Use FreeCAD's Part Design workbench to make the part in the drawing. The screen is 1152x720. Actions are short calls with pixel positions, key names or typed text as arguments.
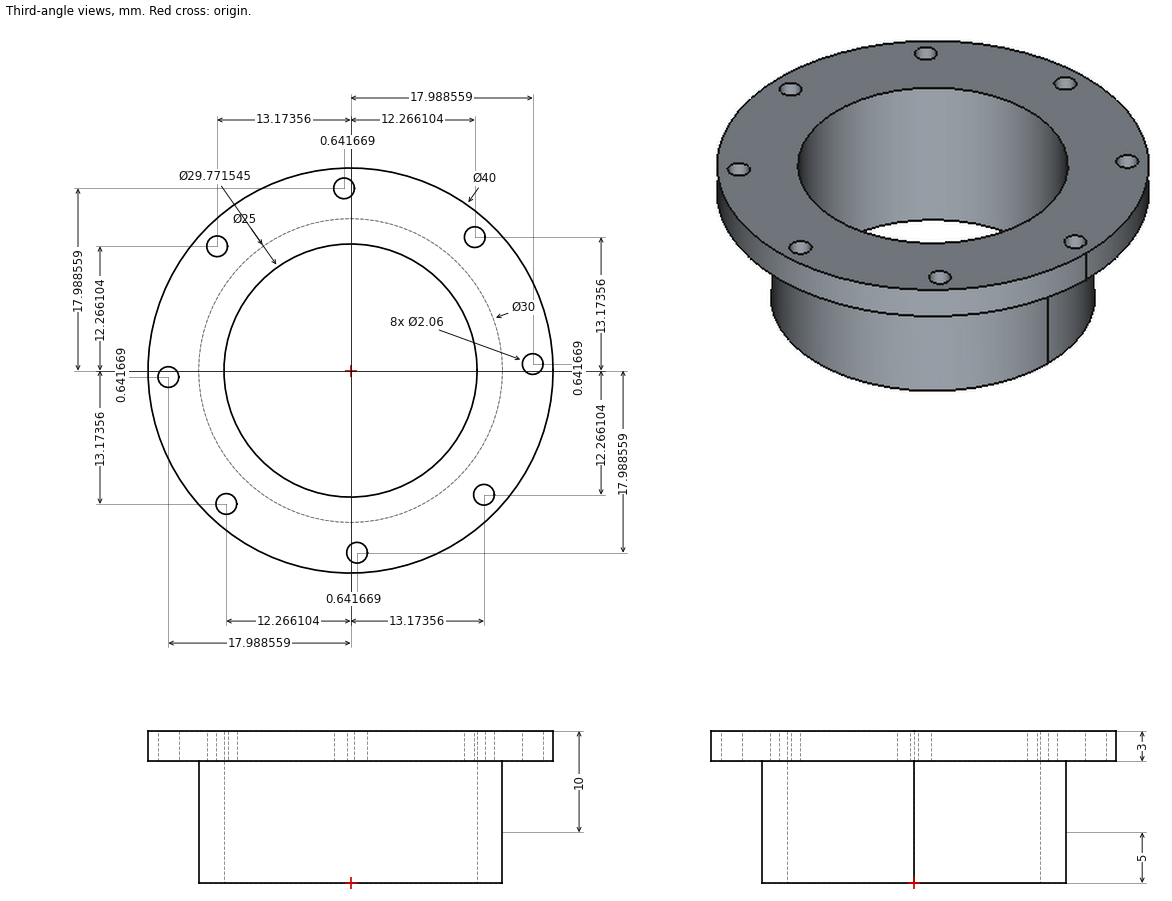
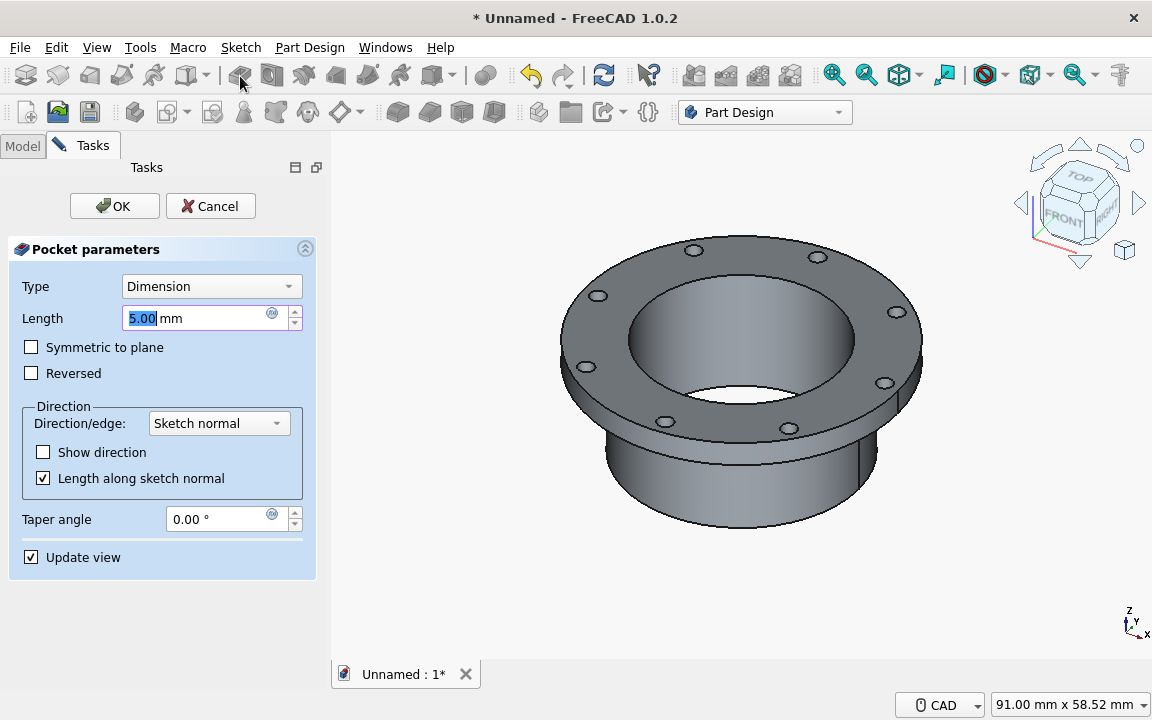
text(10)
key(Tab)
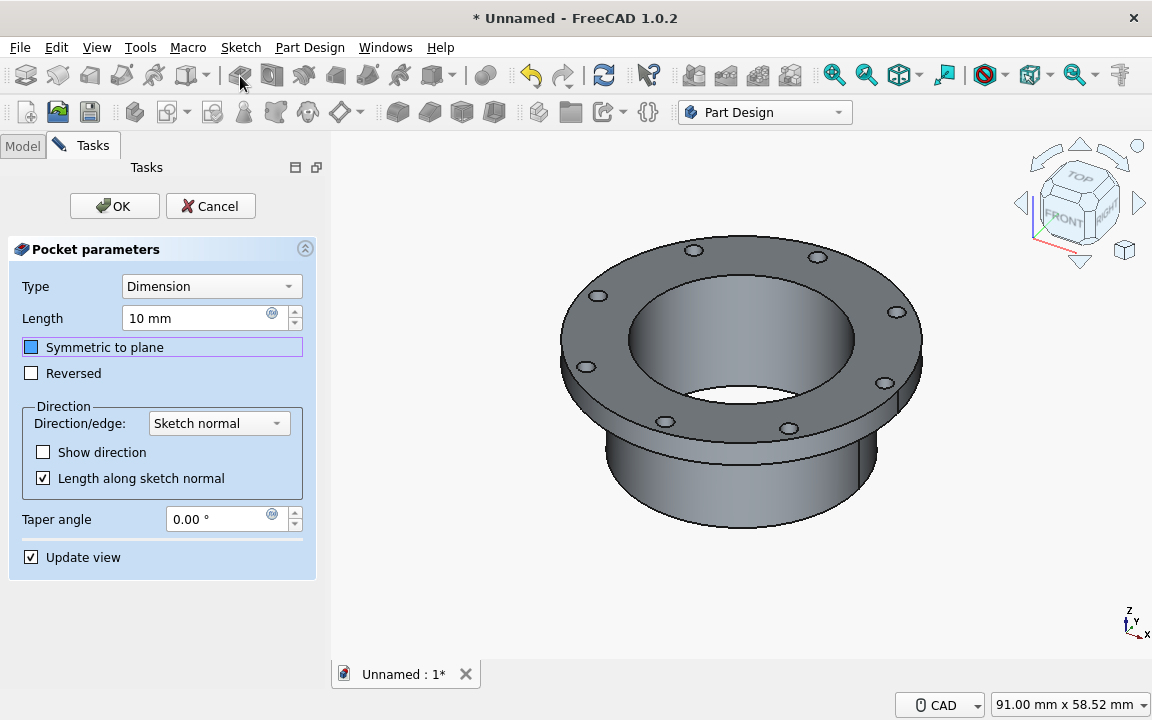
click(115, 206)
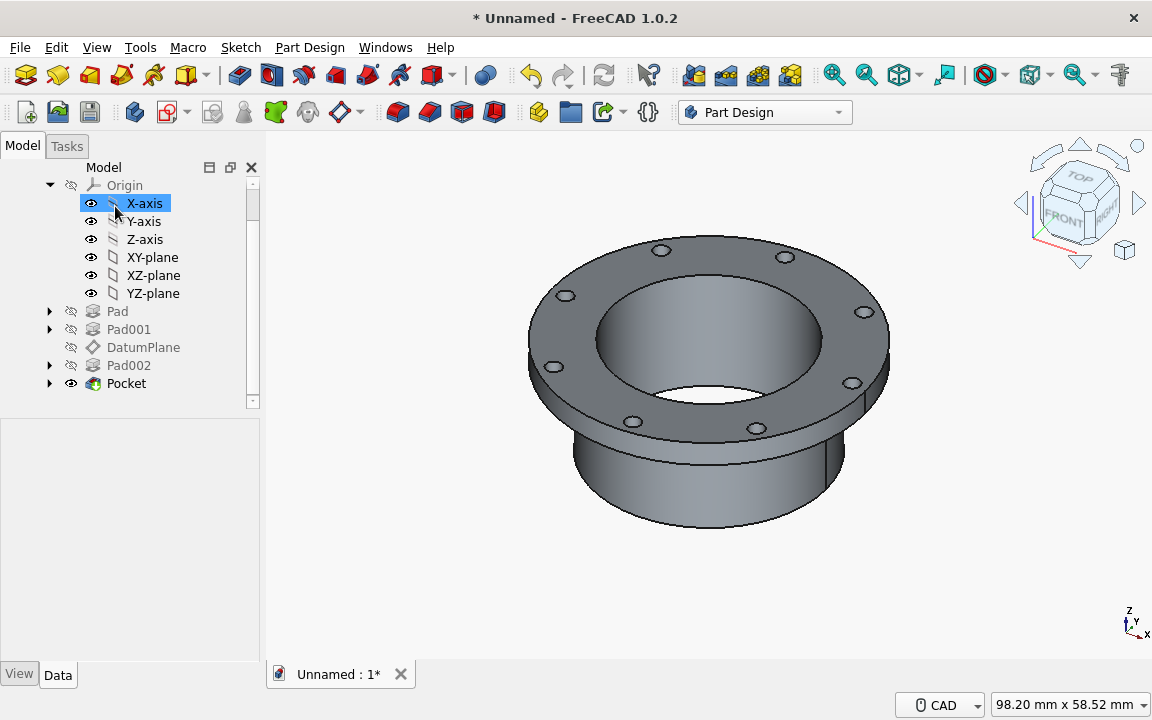
key(0)